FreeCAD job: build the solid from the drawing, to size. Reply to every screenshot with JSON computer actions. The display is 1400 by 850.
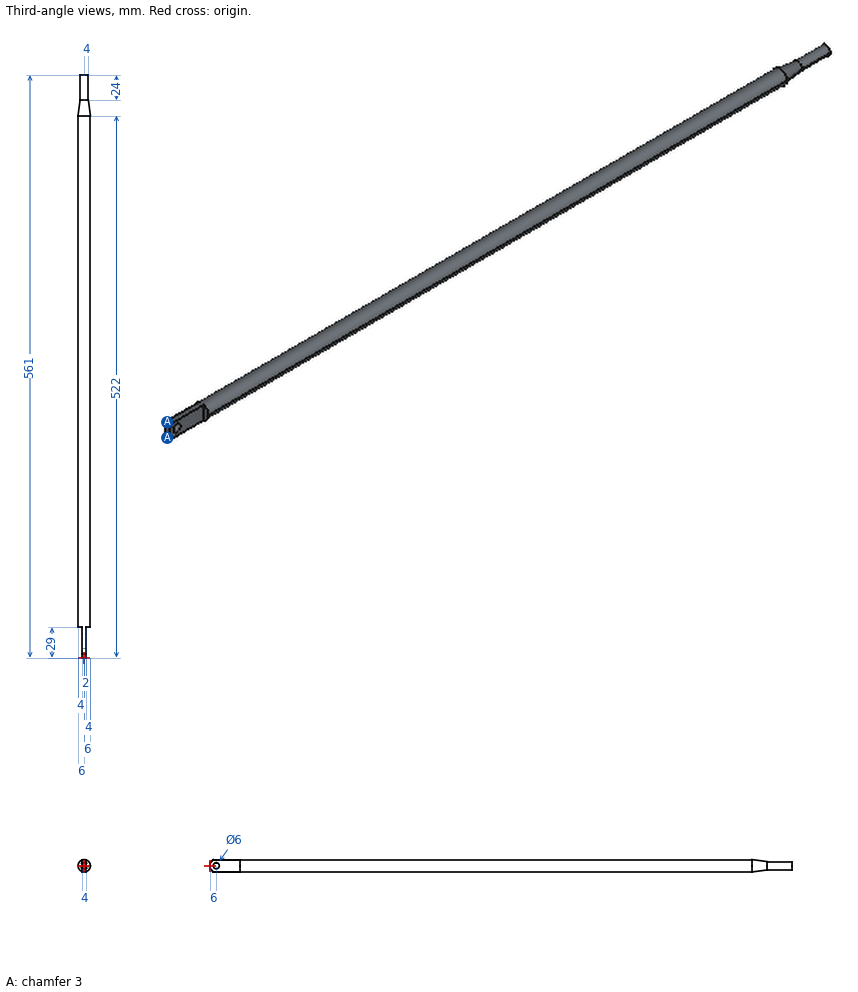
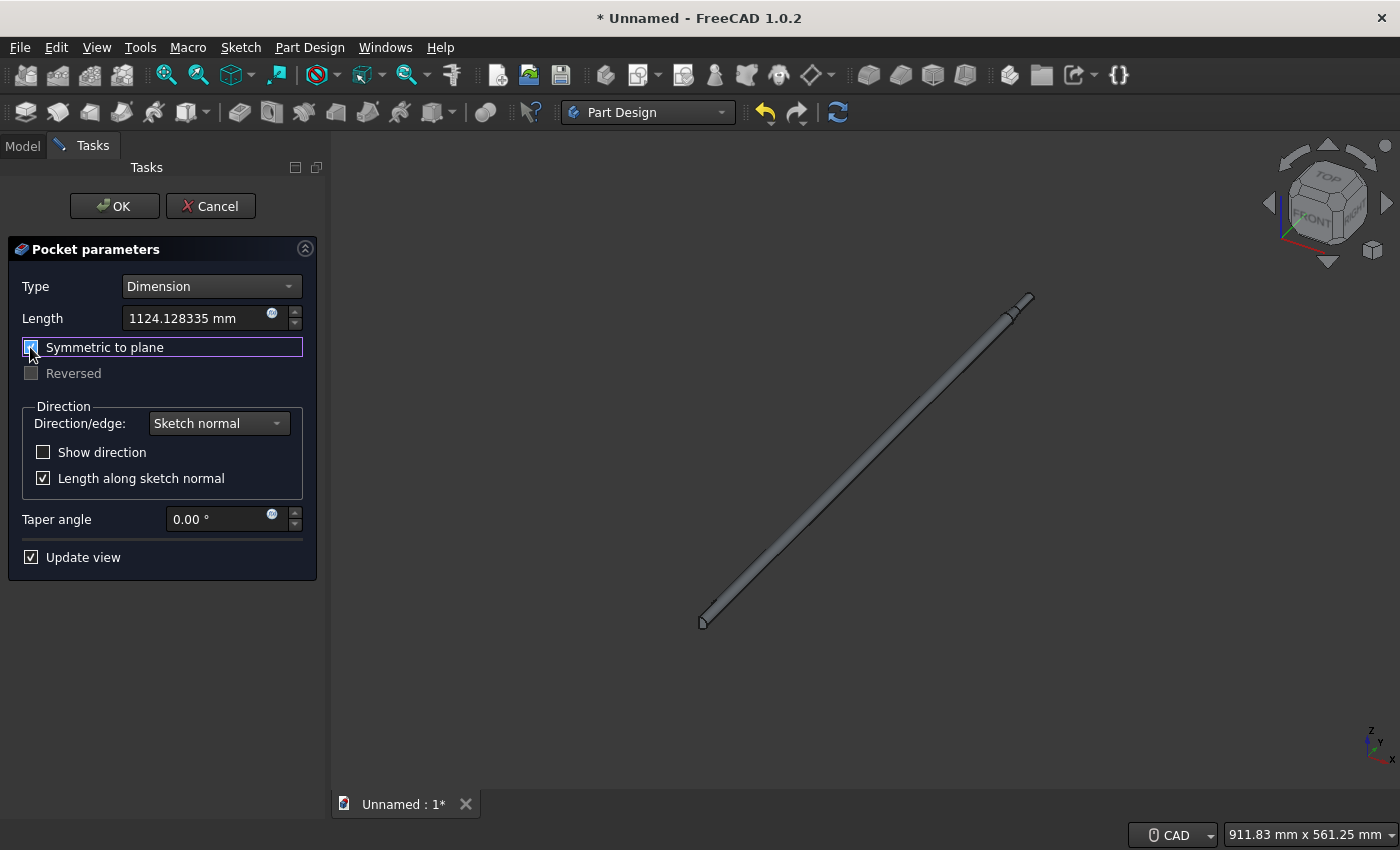
{"action": "left_click", "coordinate": [115, 206]}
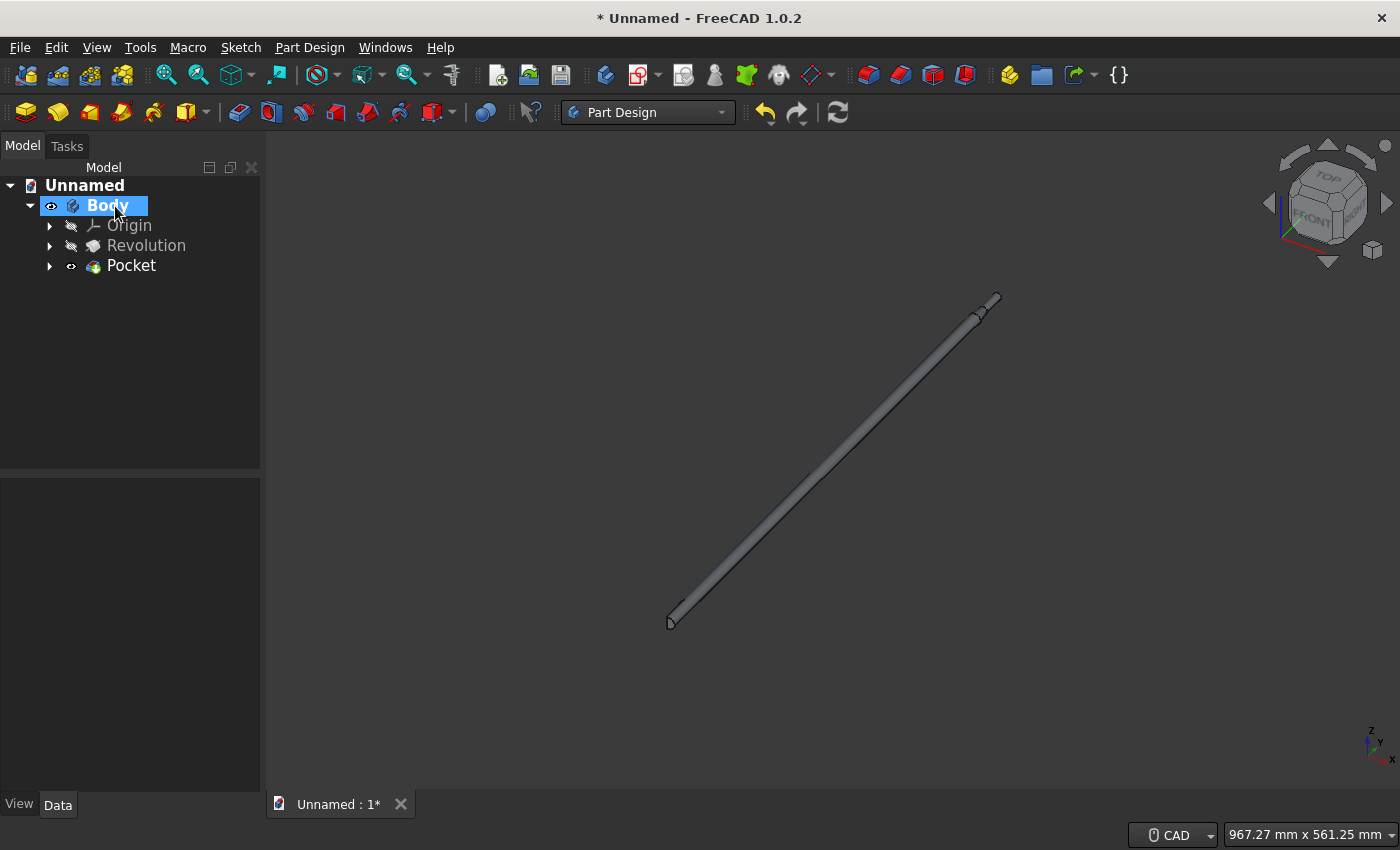
{"action": "left_click", "coordinate": [638, 76]}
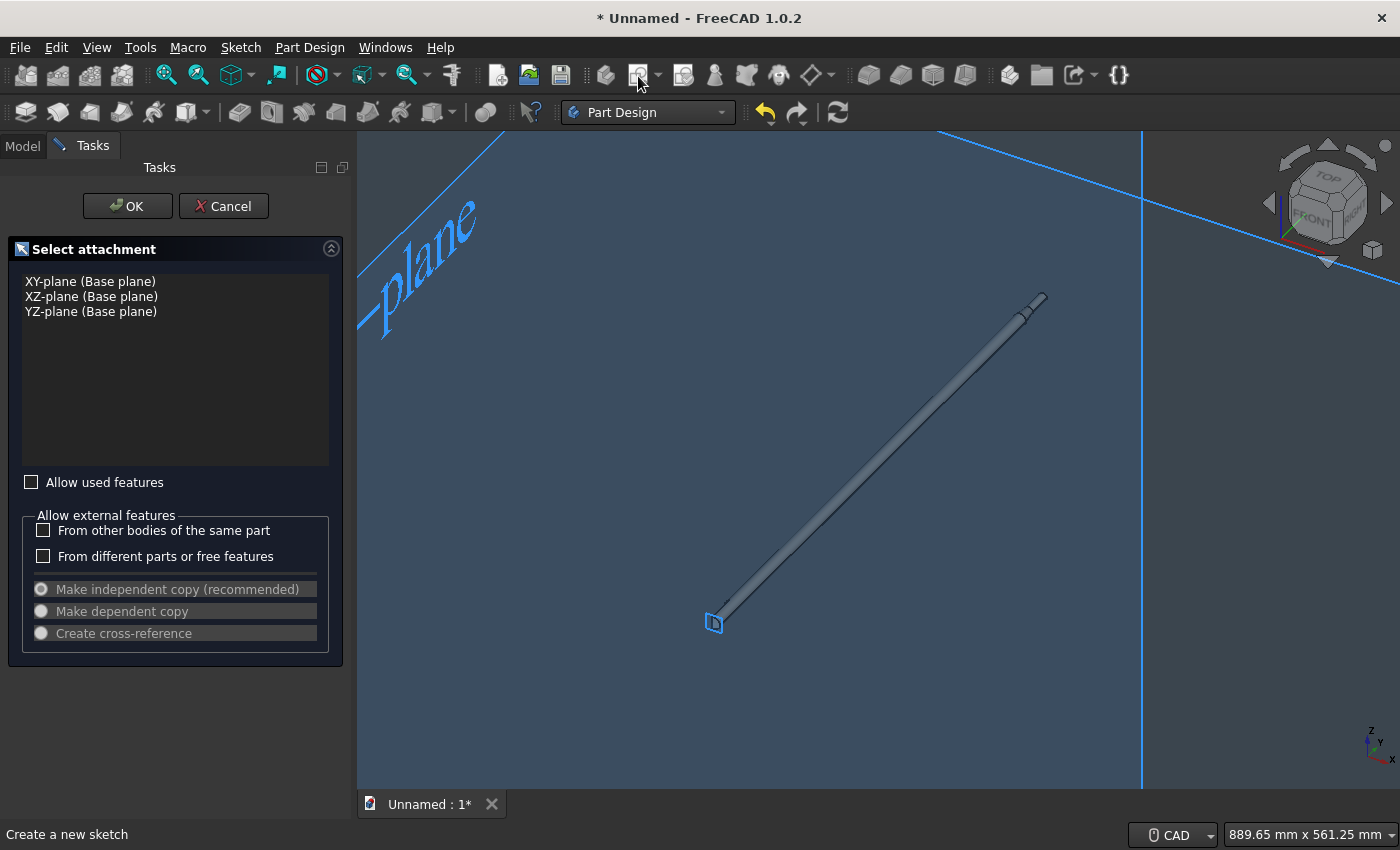
{"action": "left_click", "coordinate": [82, 282]}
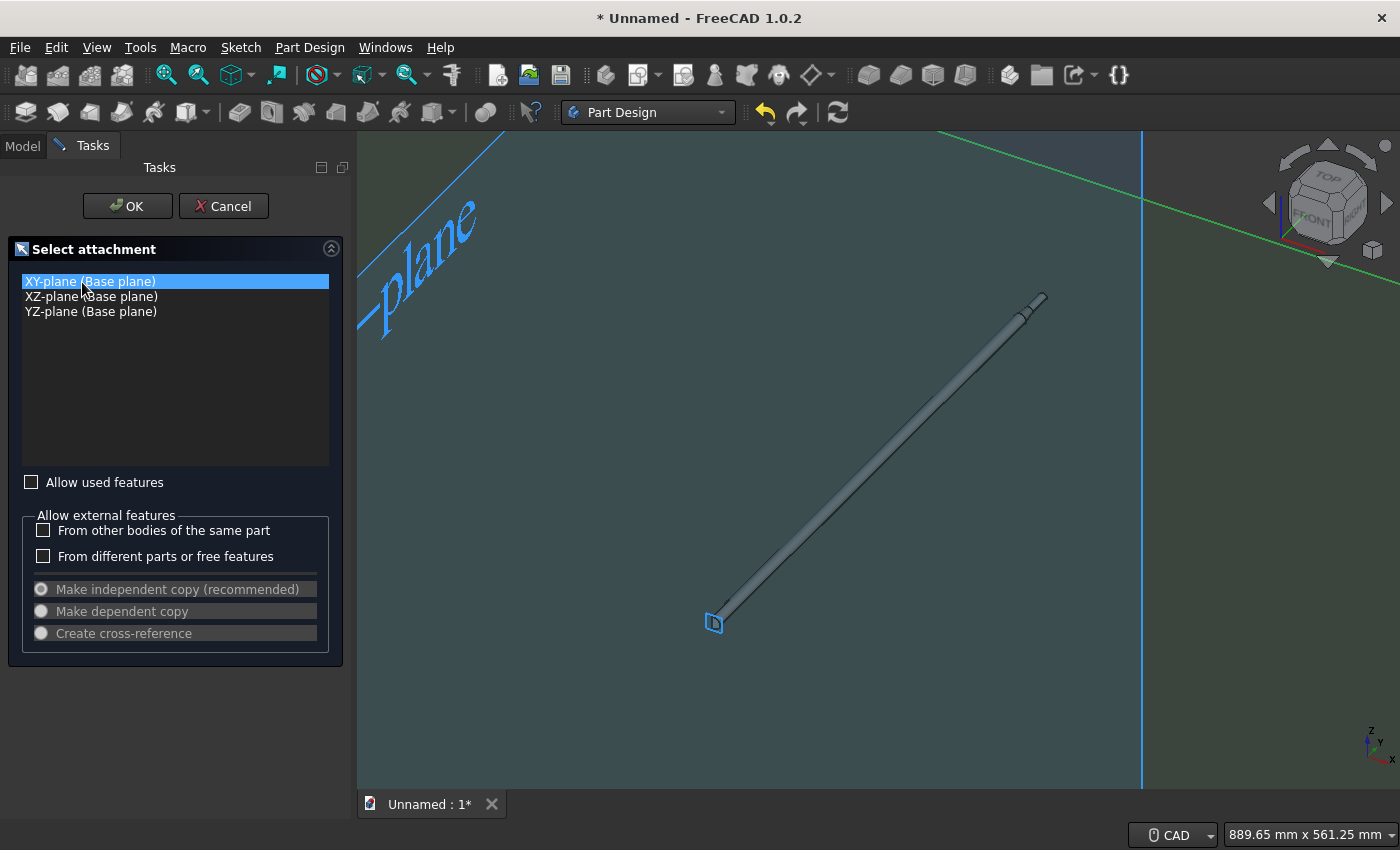
{"action": "left_click", "coordinate": [128, 206]}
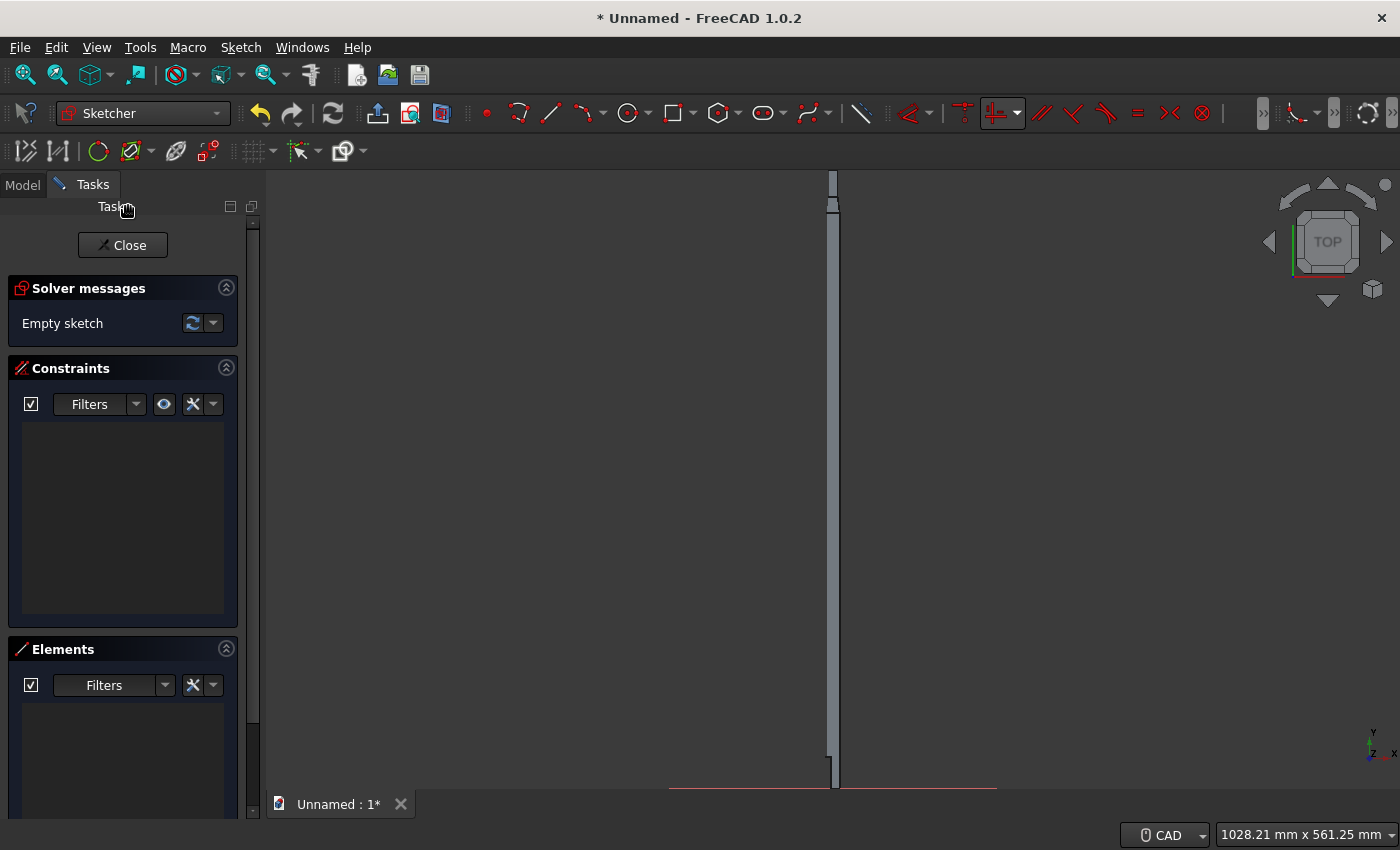
{"action": "left_click", "coordinate": [442, 114]}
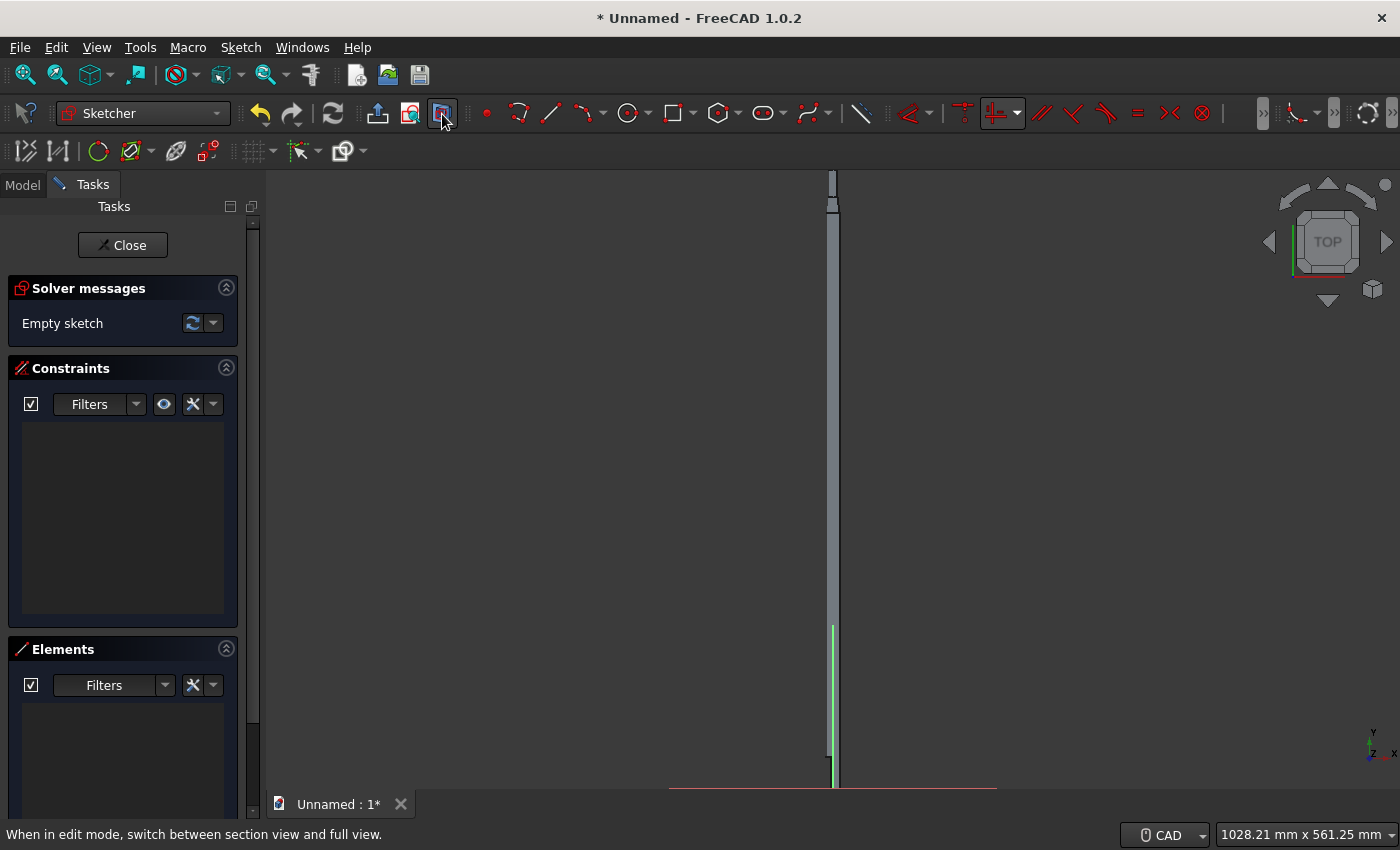
{"action": "scroll", "coordinate": [764, 480], "scroll_direction": "down", "scroll_amount": 5}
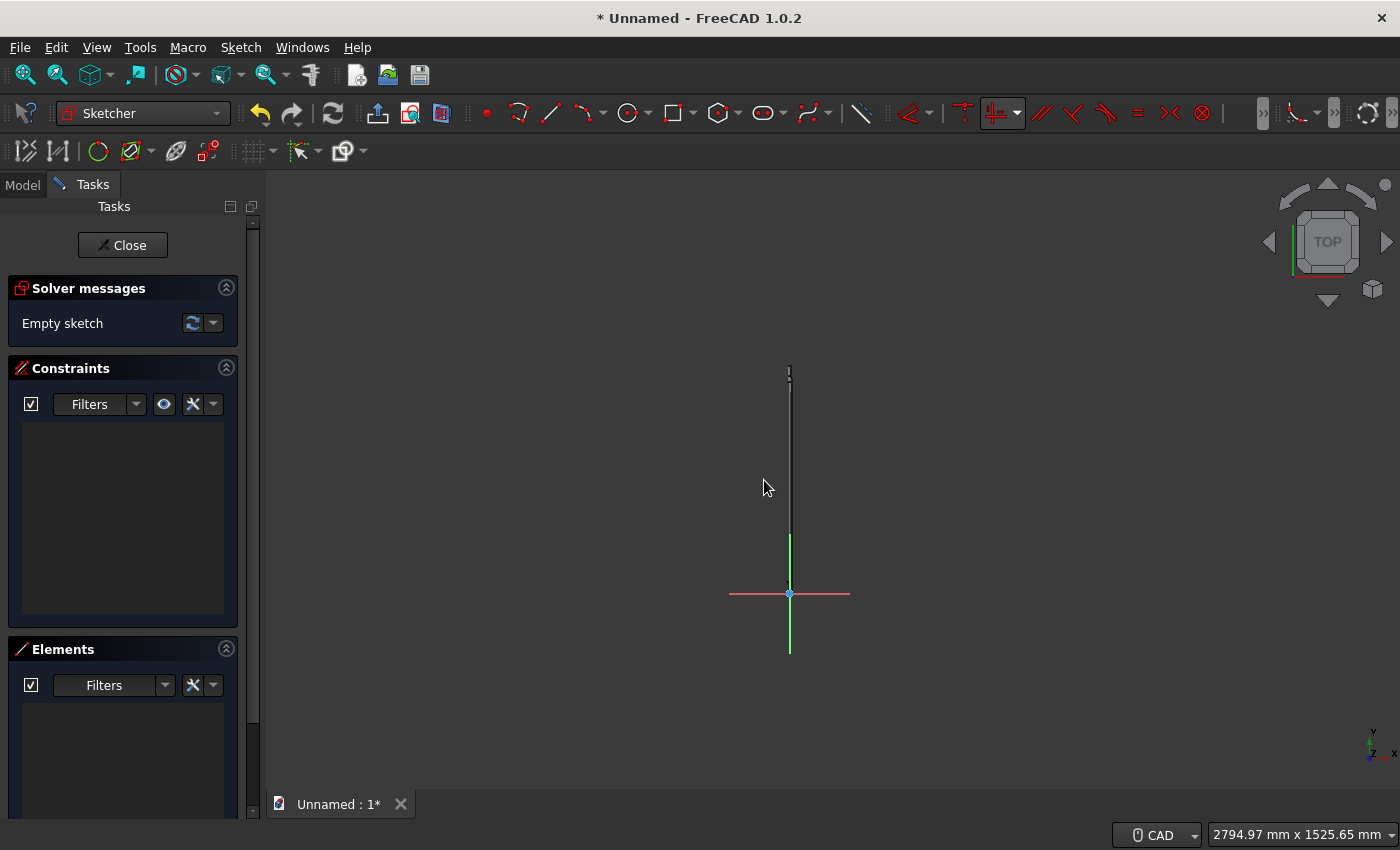
{"action": "scroll", "coordinate": [792, 594], "scroll_direction": "up", "scroll_amount": 15}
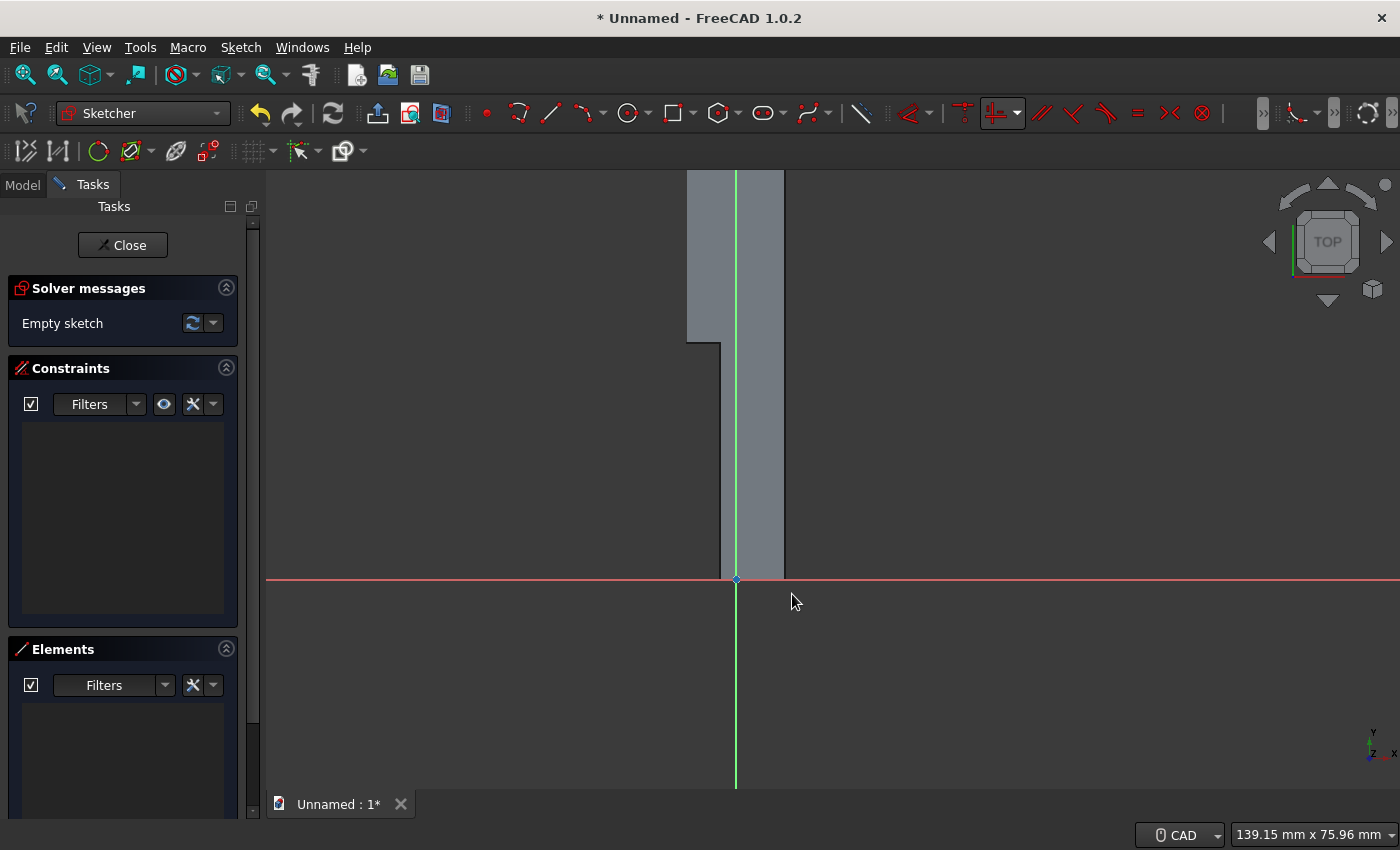
{"action": "scroll", "coordinate": [756, 440], "scroll_direction": "up", "scroll_amount": 3}